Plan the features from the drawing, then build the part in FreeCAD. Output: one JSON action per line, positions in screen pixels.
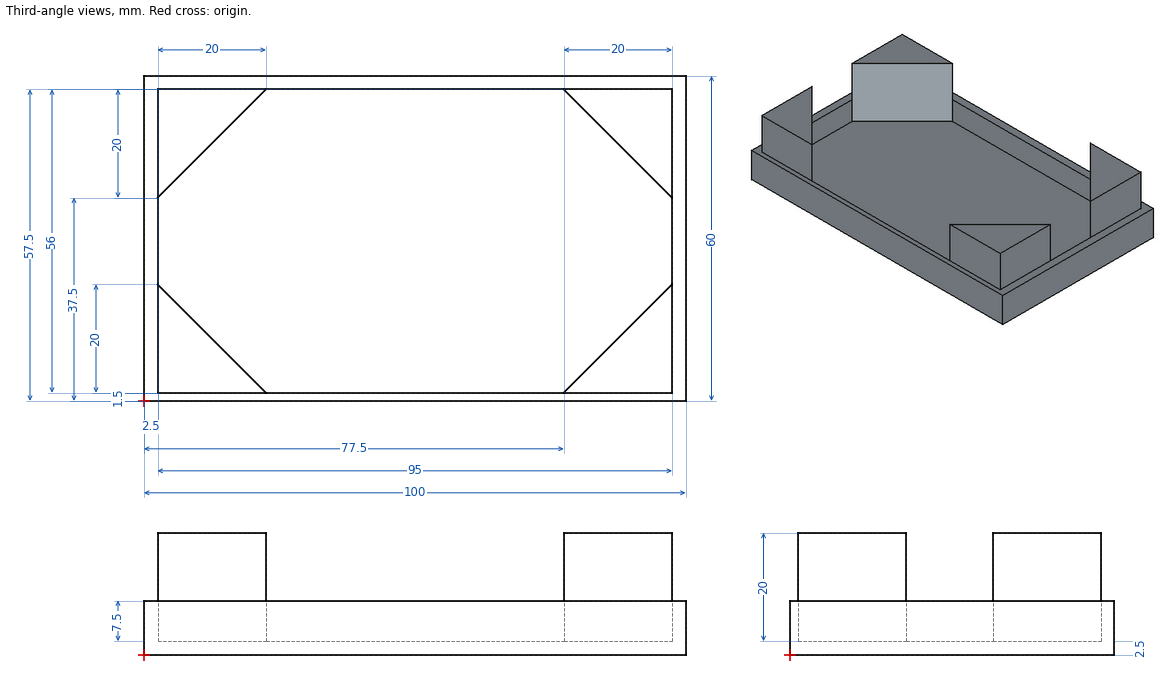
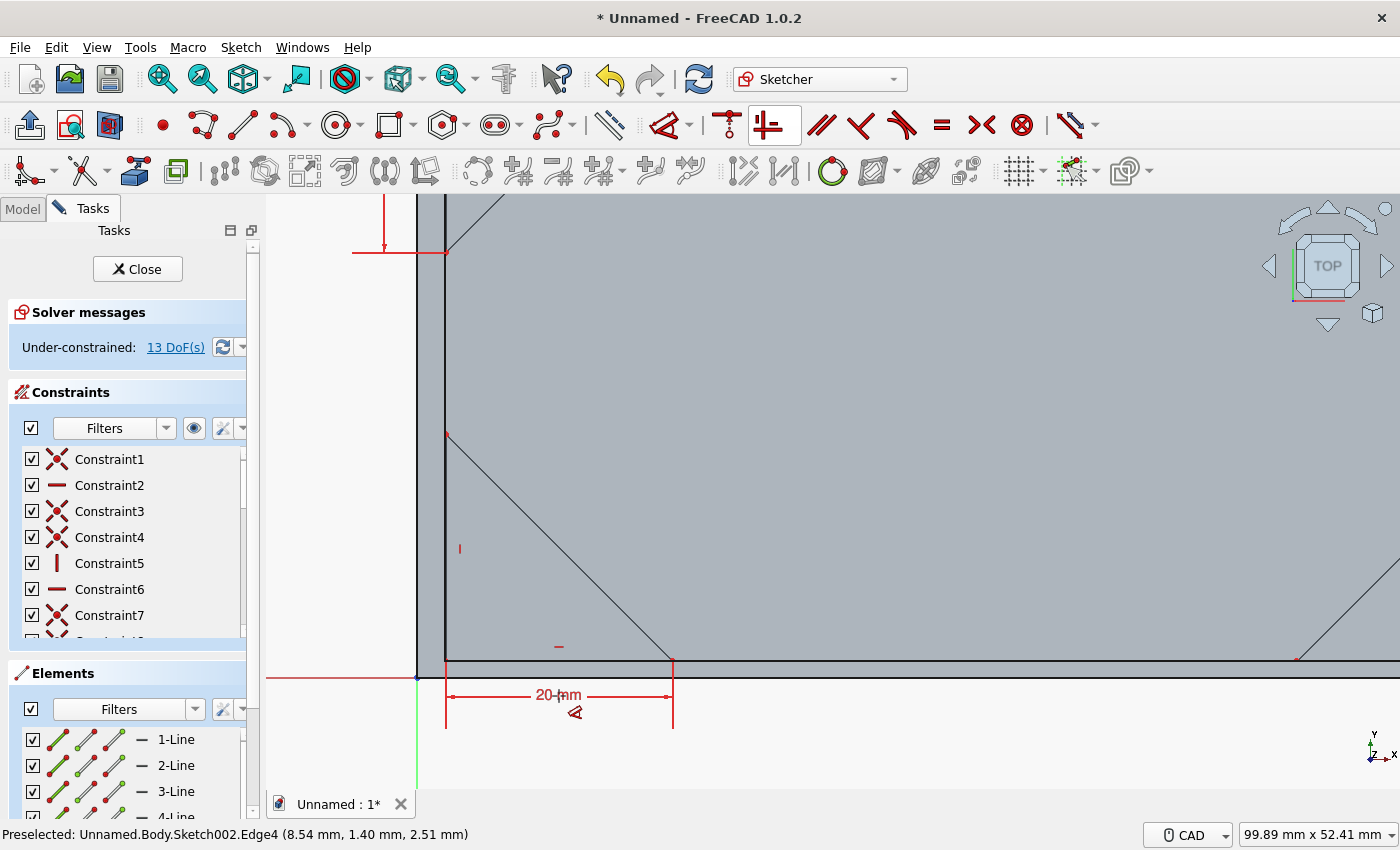
{"action": "left_click", "coordinate": [446, 503]}
{"action": "left_click", "coordinate": [480, 548]}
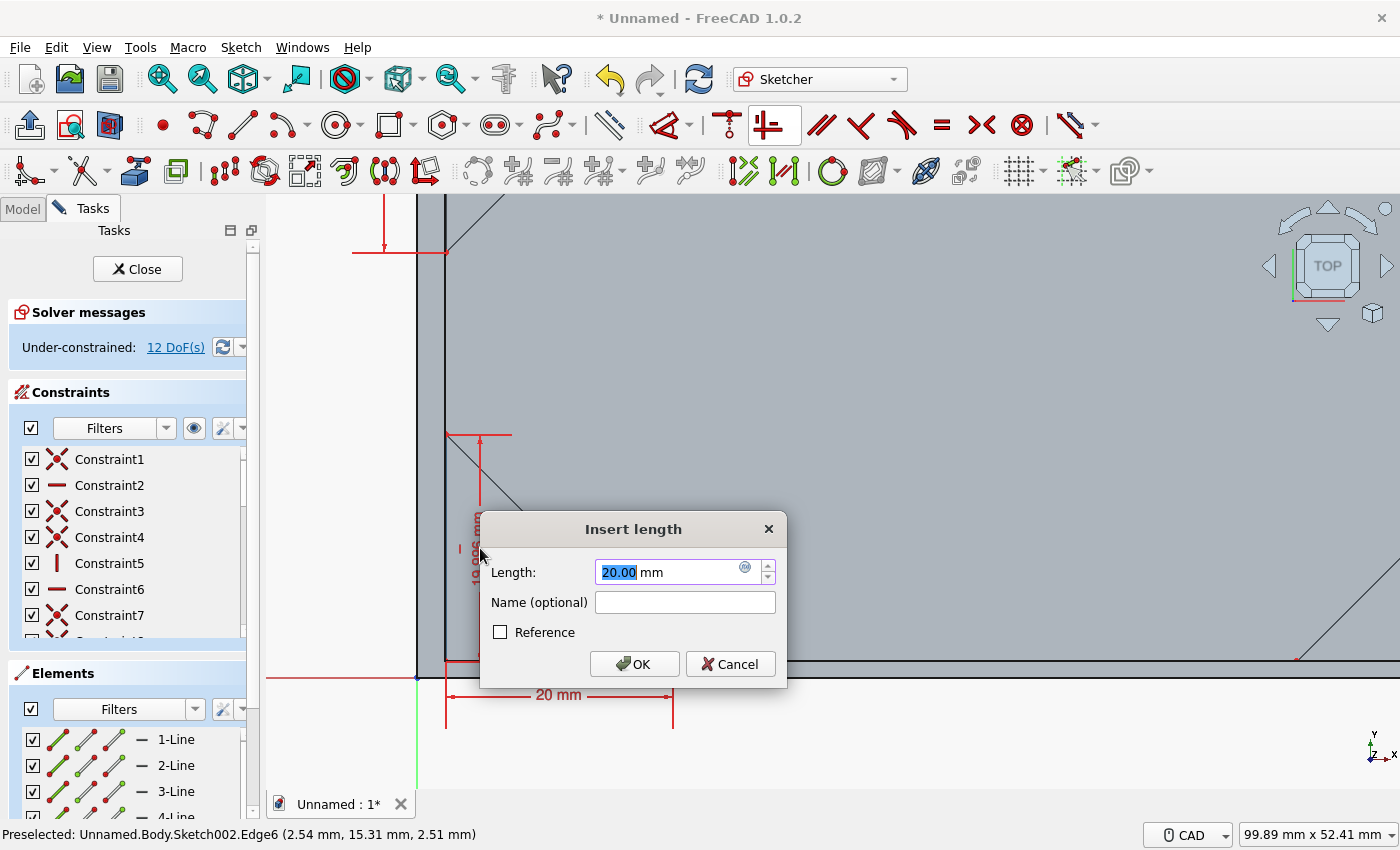
{"action": "type", "text": "20"}
{"action": "key", "text": "Return"}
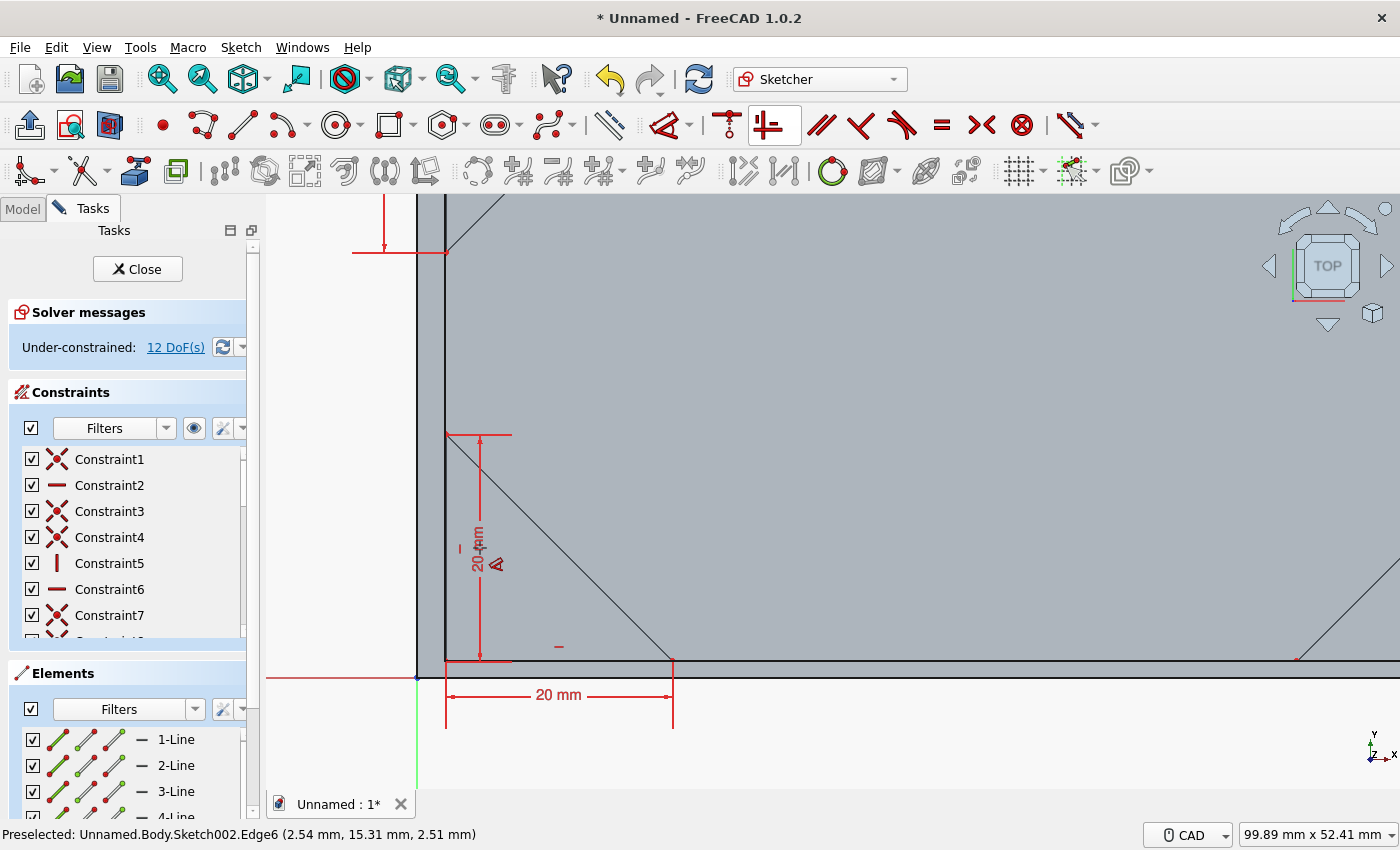
{"action": "scroll", "coordinate": [514, 662], "scroll_direction": "down", "scroll_amount": 3}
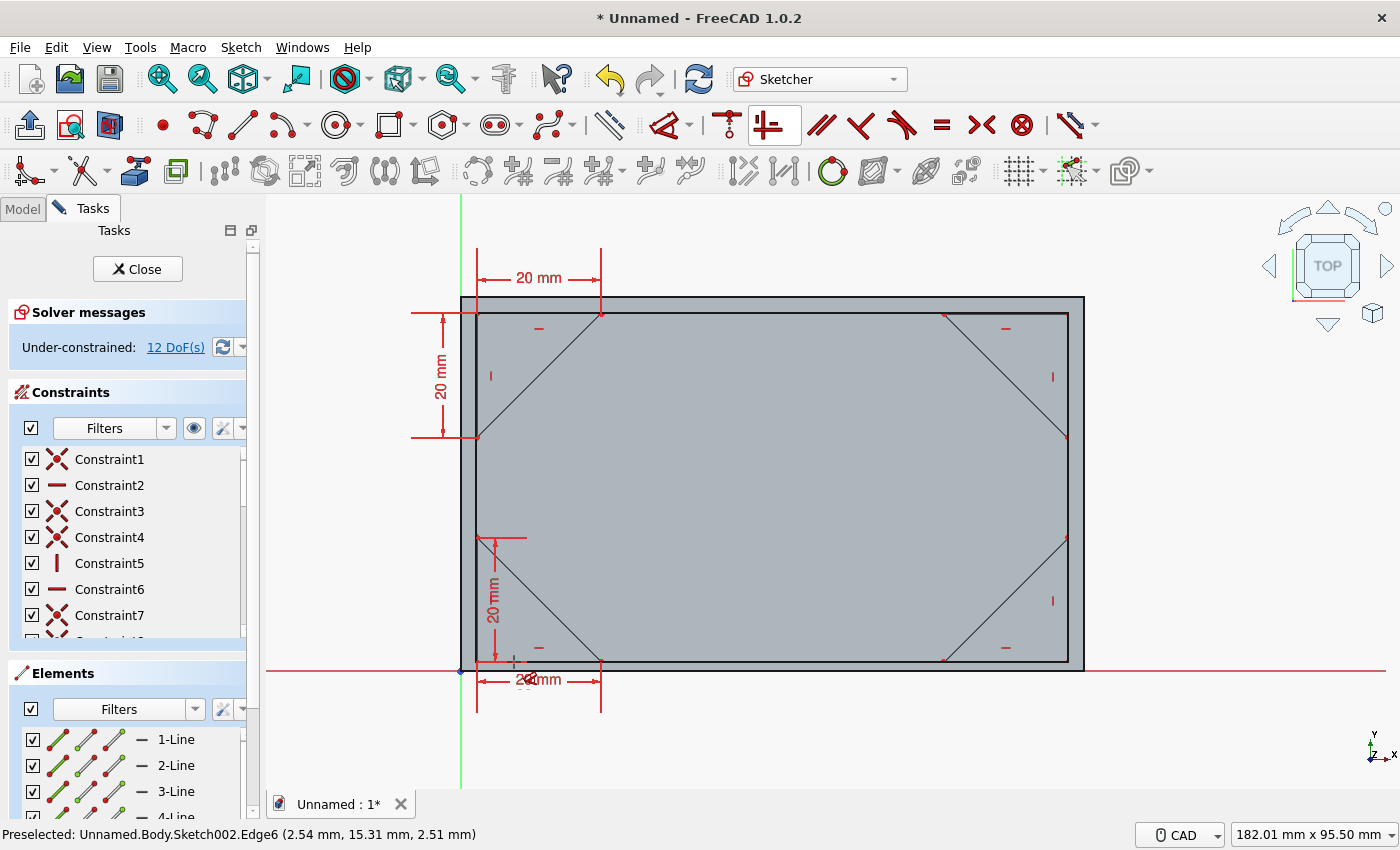
{"action": "left_click", "coordinate": [1068, 401]}
{"action": "left_click", "coordinate": [1102, 376]}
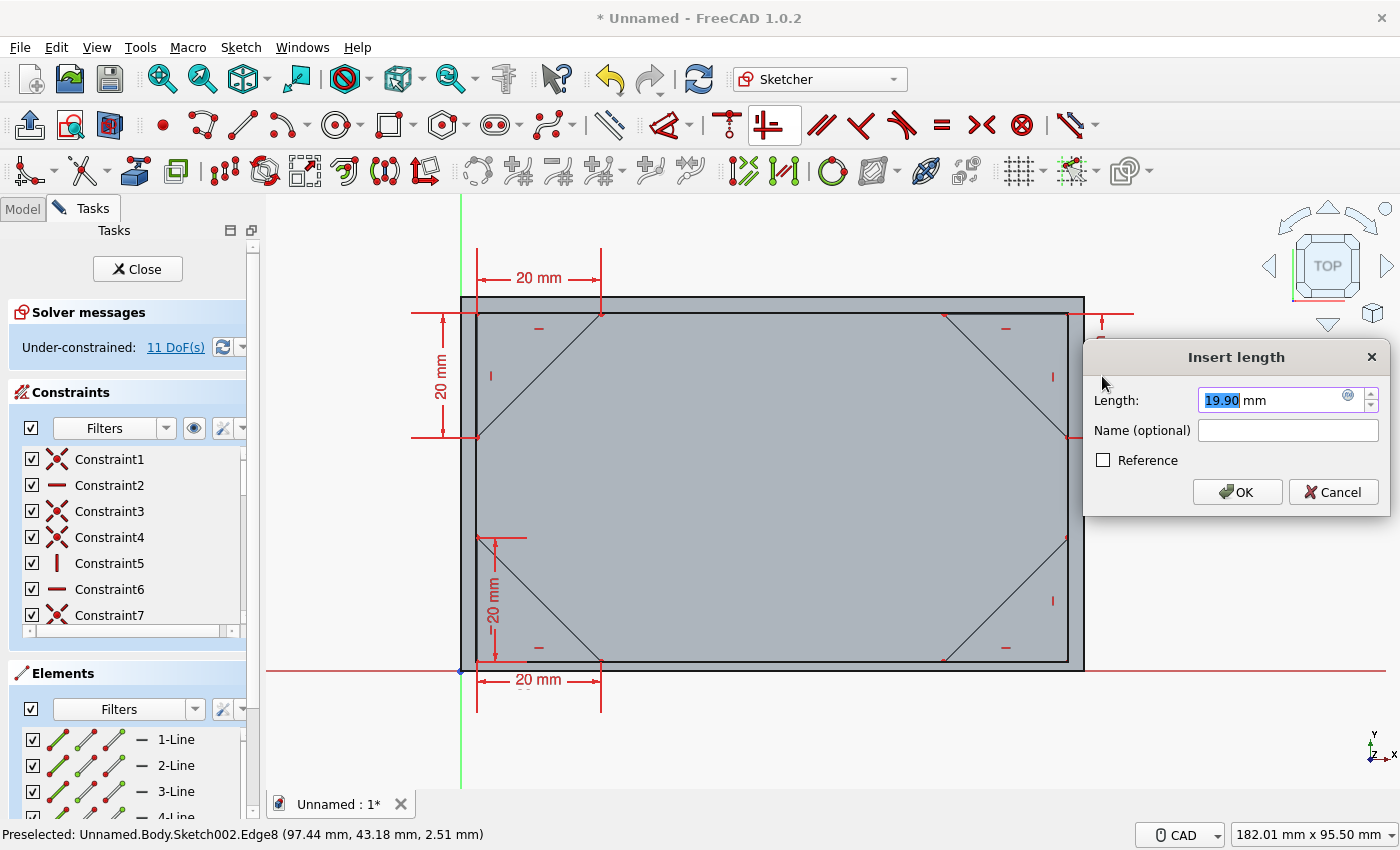
{"action": "type", "text": "20"}
{"action": "key", "text": "Return"}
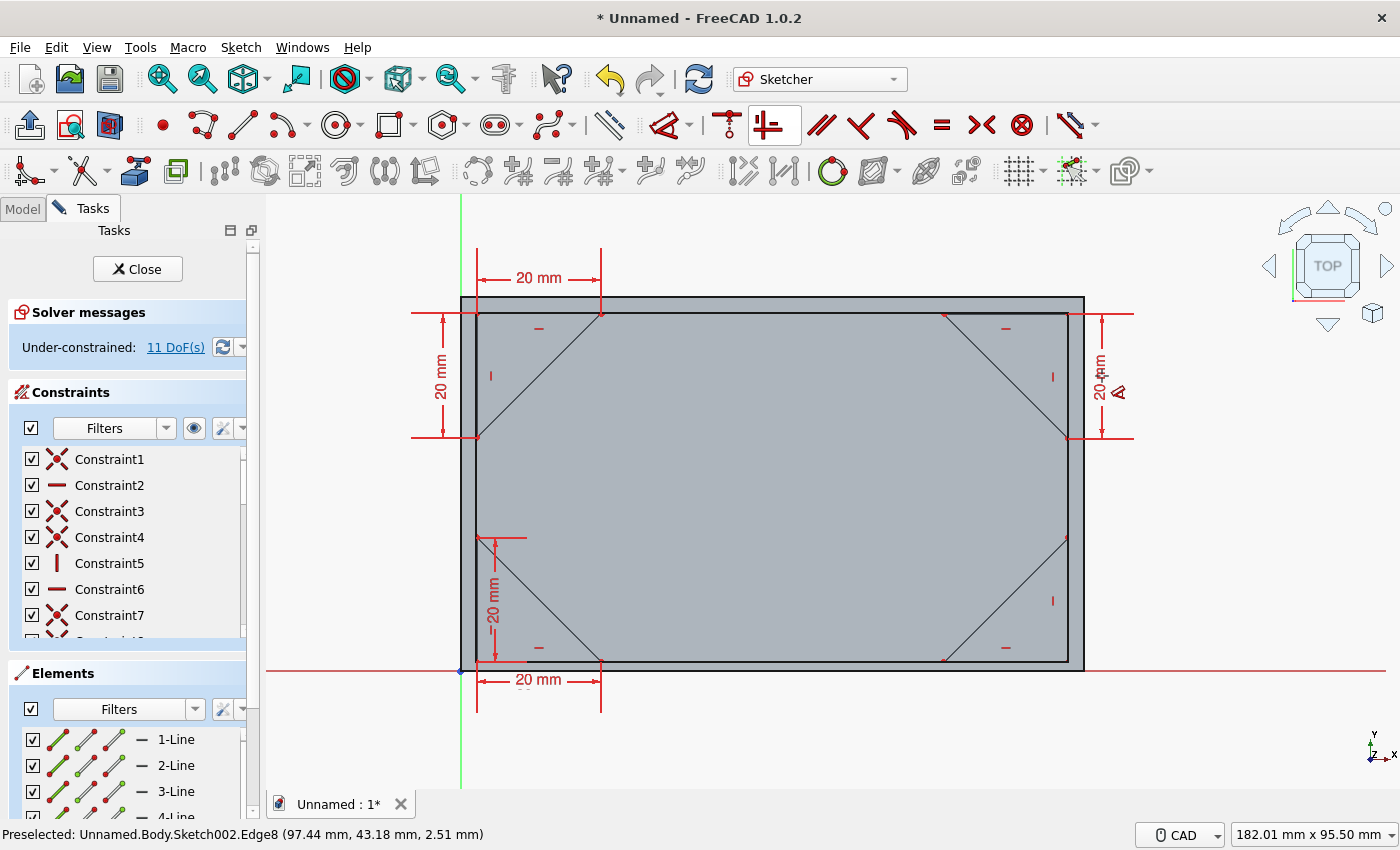
{"action": "left_click", "coordinate": [1031, 314]}
{"action": "left_click", "coordinate": [1006, 280]}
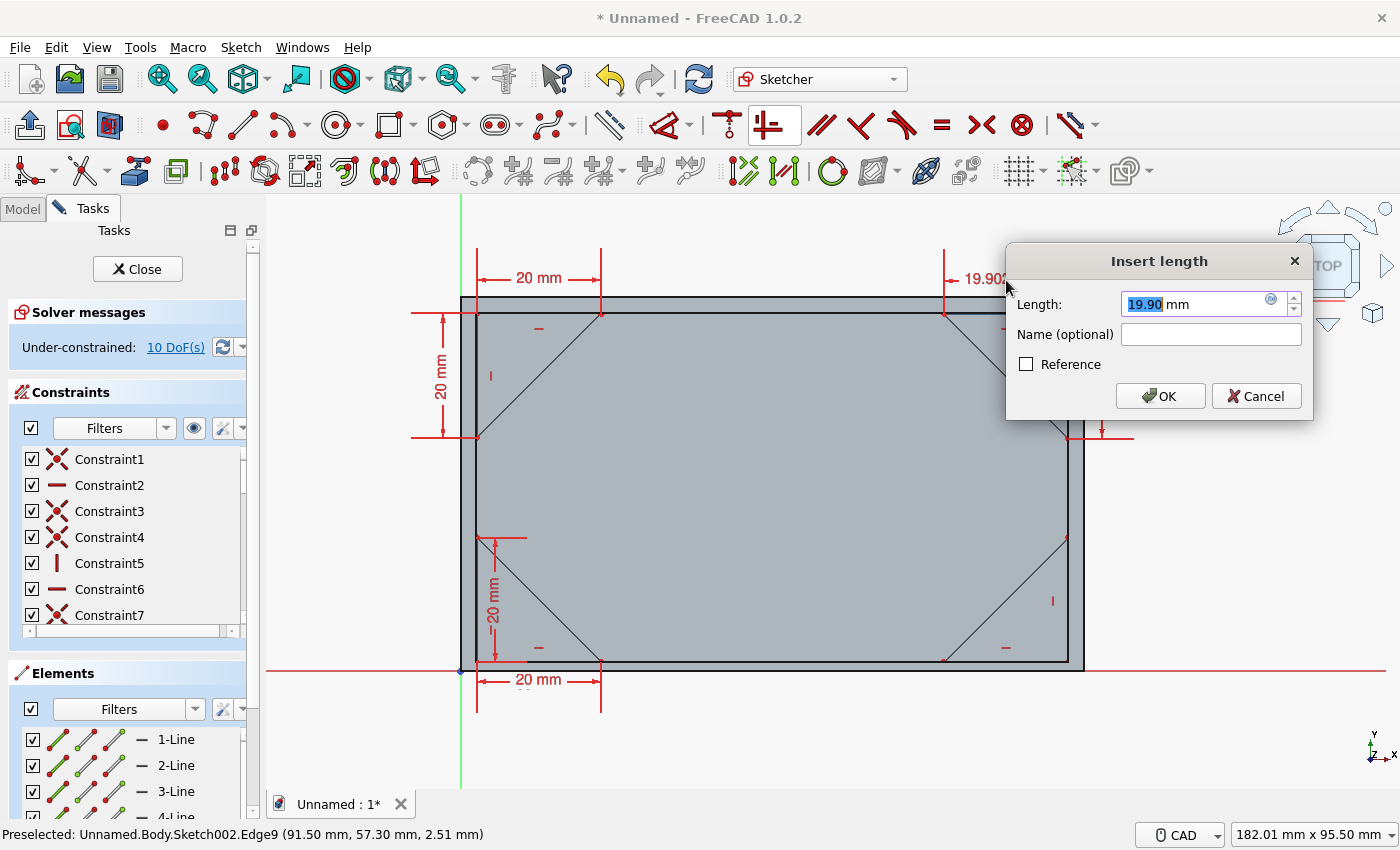
{"action": "type", "text": "20"}
{"action": "key", "text": "Return"}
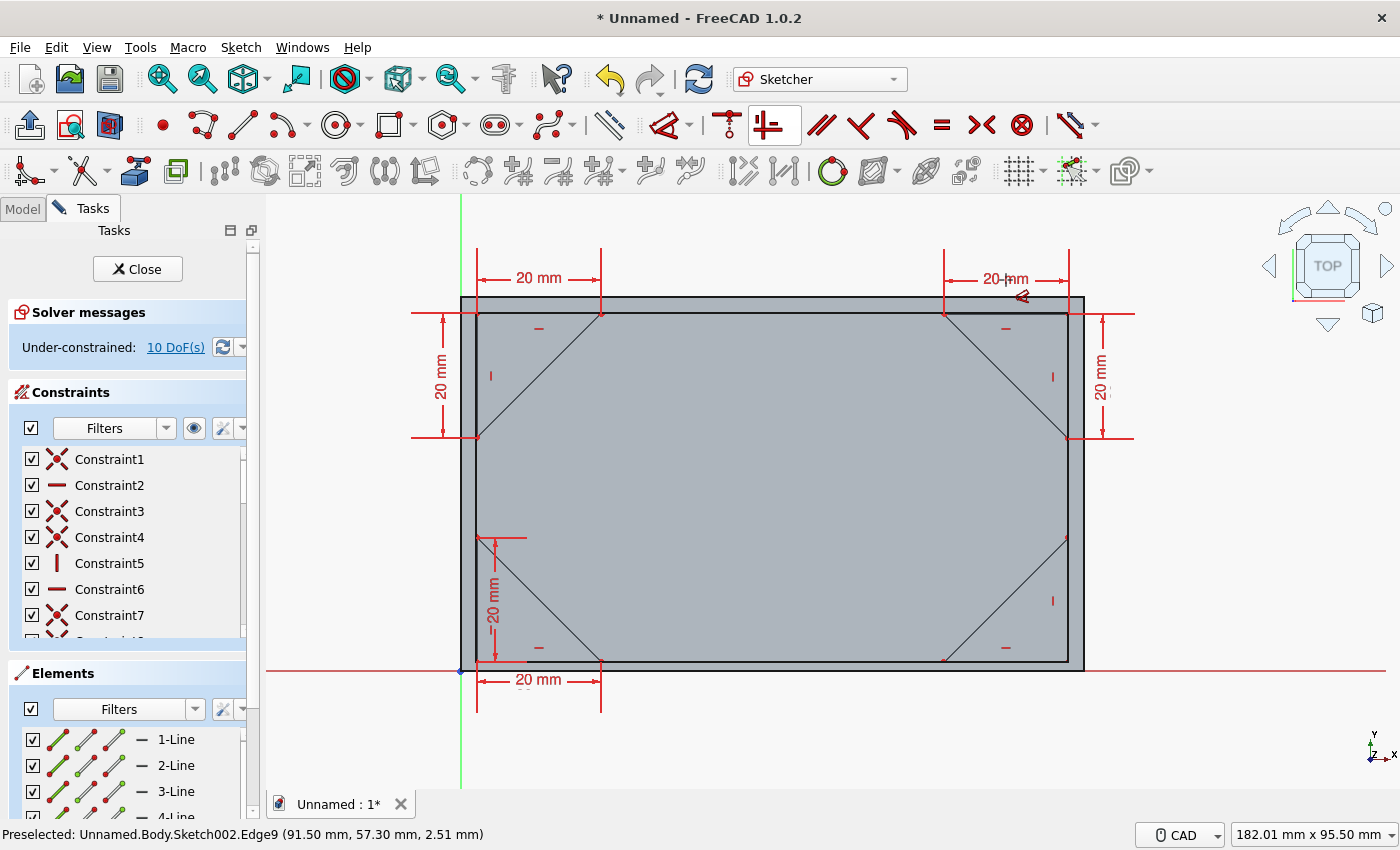
{"action": "scroll", "coordinate": [981, 662], "scroll_direction": "up", "scroll_amount": 3}